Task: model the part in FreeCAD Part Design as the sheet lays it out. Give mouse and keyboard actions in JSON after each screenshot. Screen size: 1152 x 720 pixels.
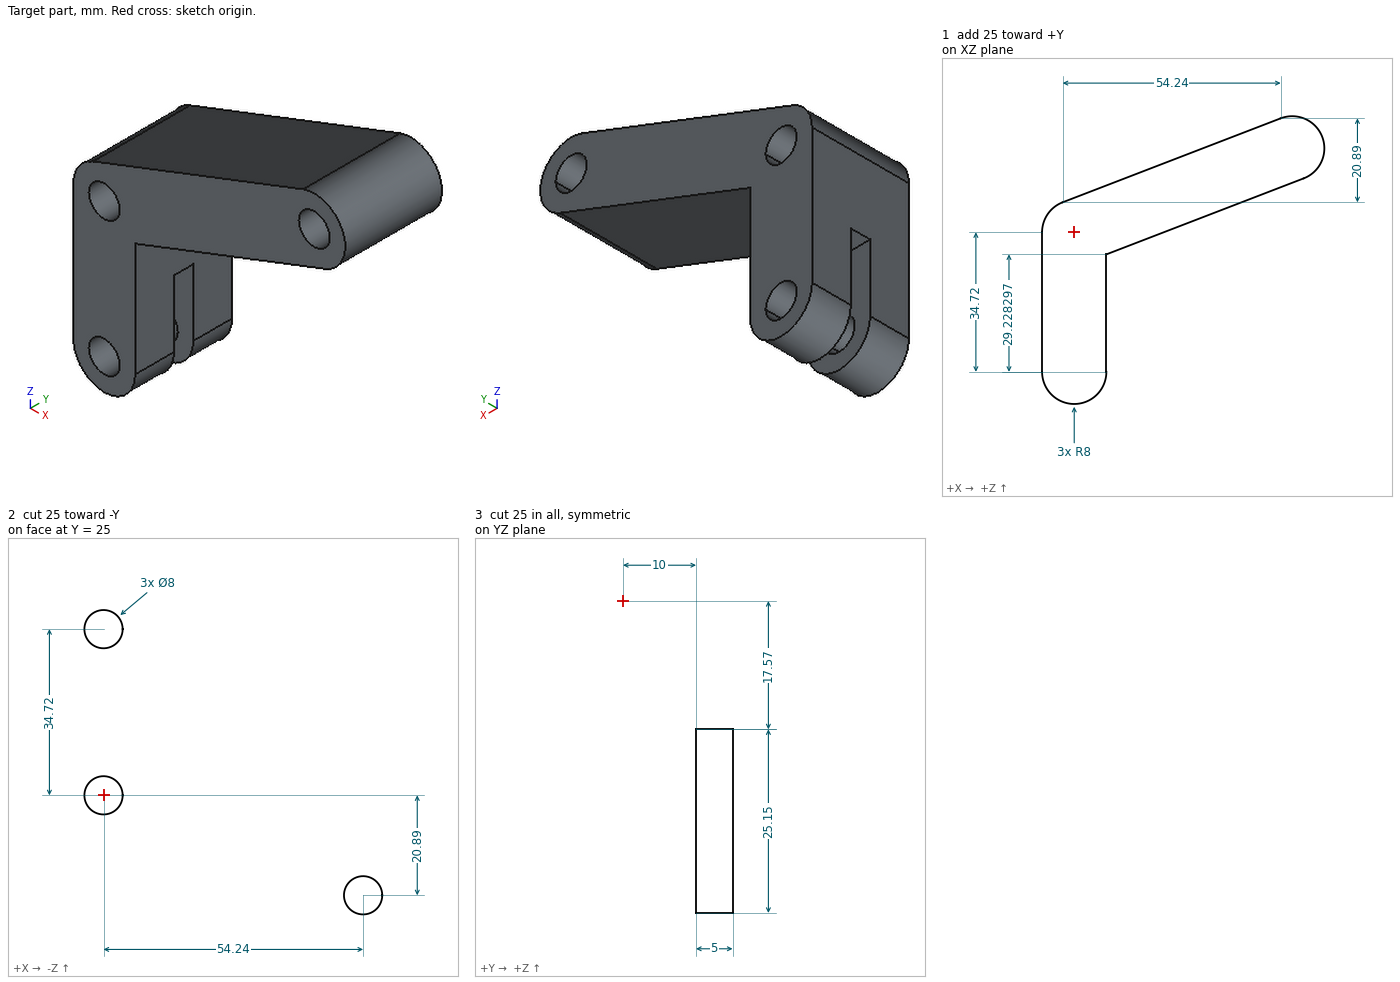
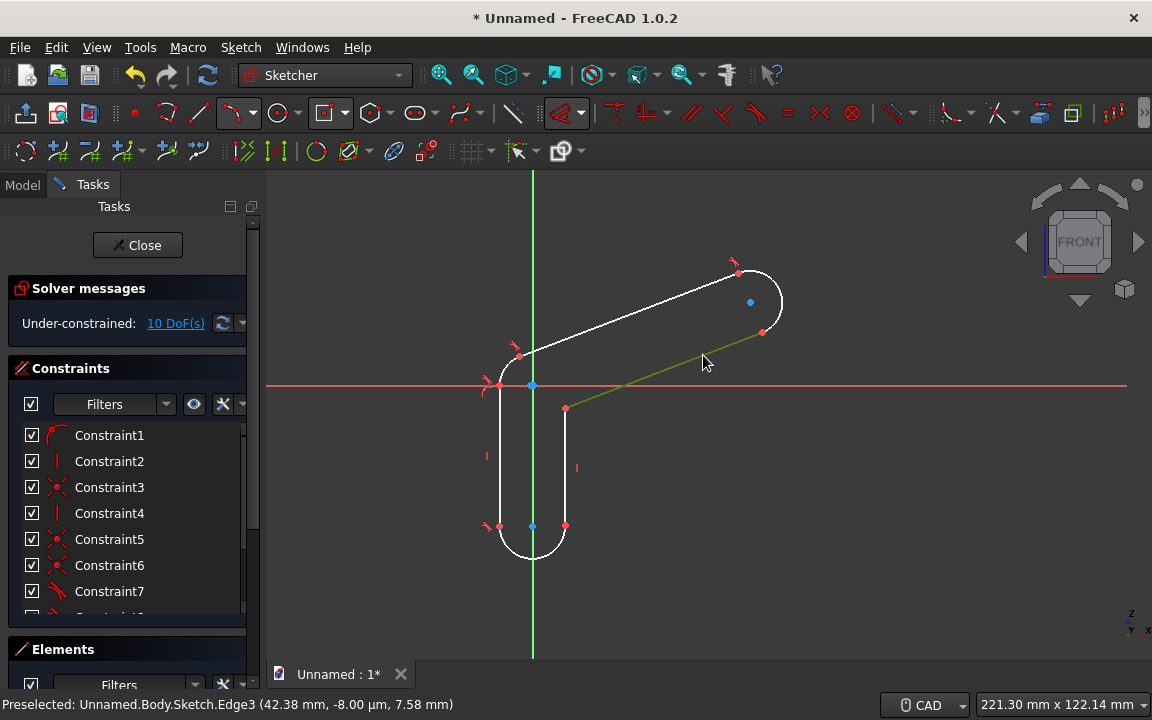
{"action": "left_click", "coordinate": [781, 311]}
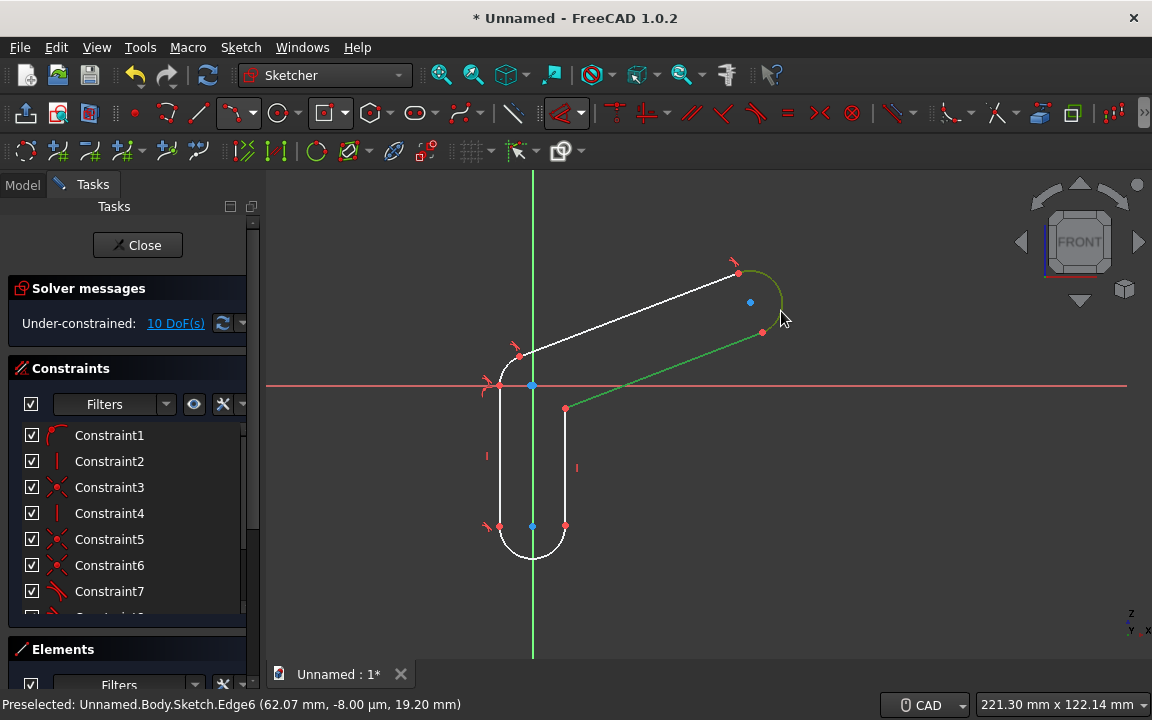
{"action": "left_click", "coordinate": [756, 114]}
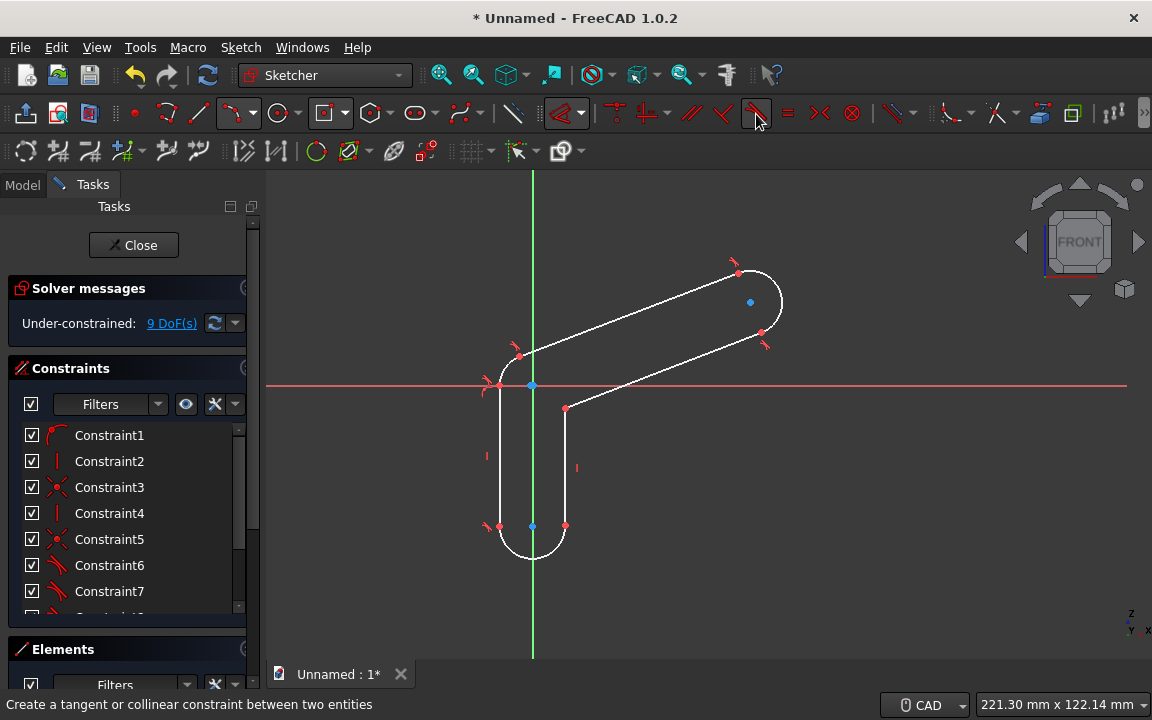
{"action": "left_click", "coordinate": [565, 444]}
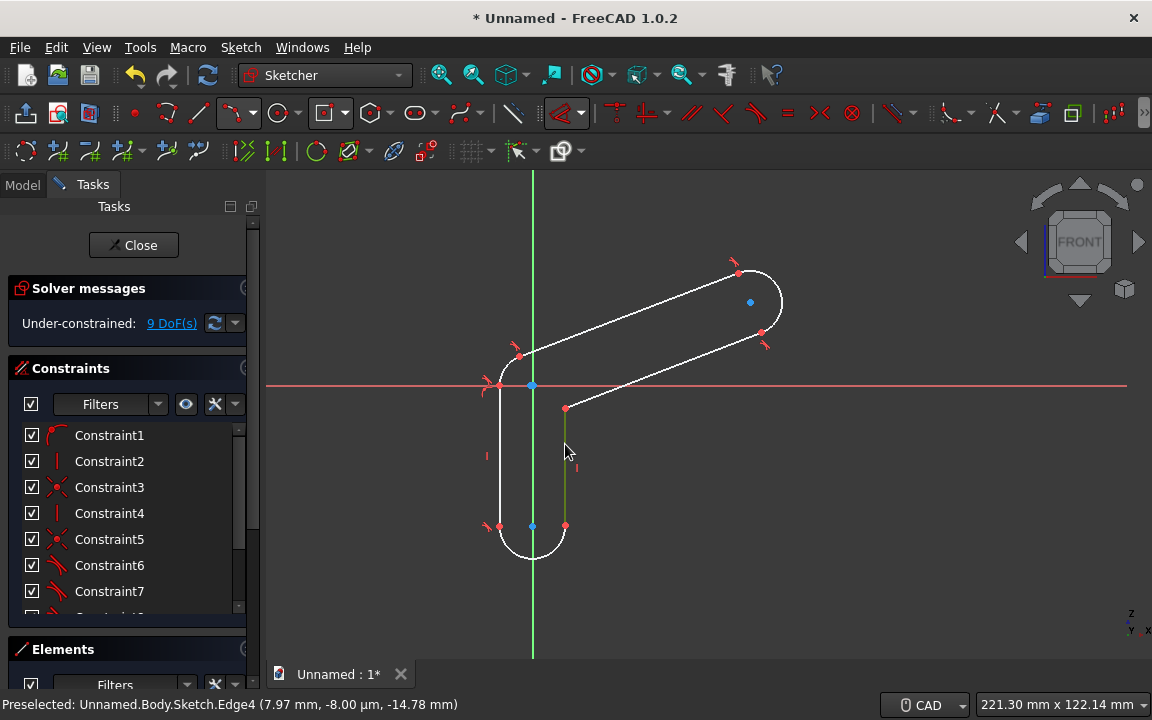
{"action": "left_click", "coordinate": [513, 553]}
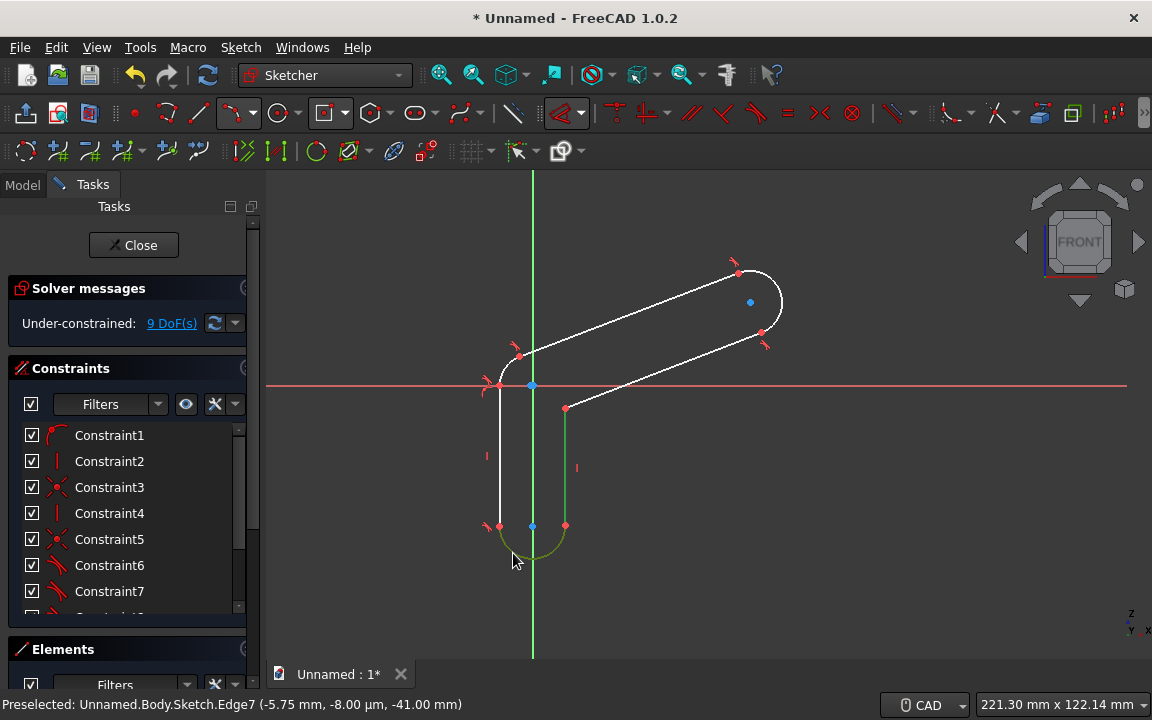
{"action": "left_click", "coordinate": [756, 114]}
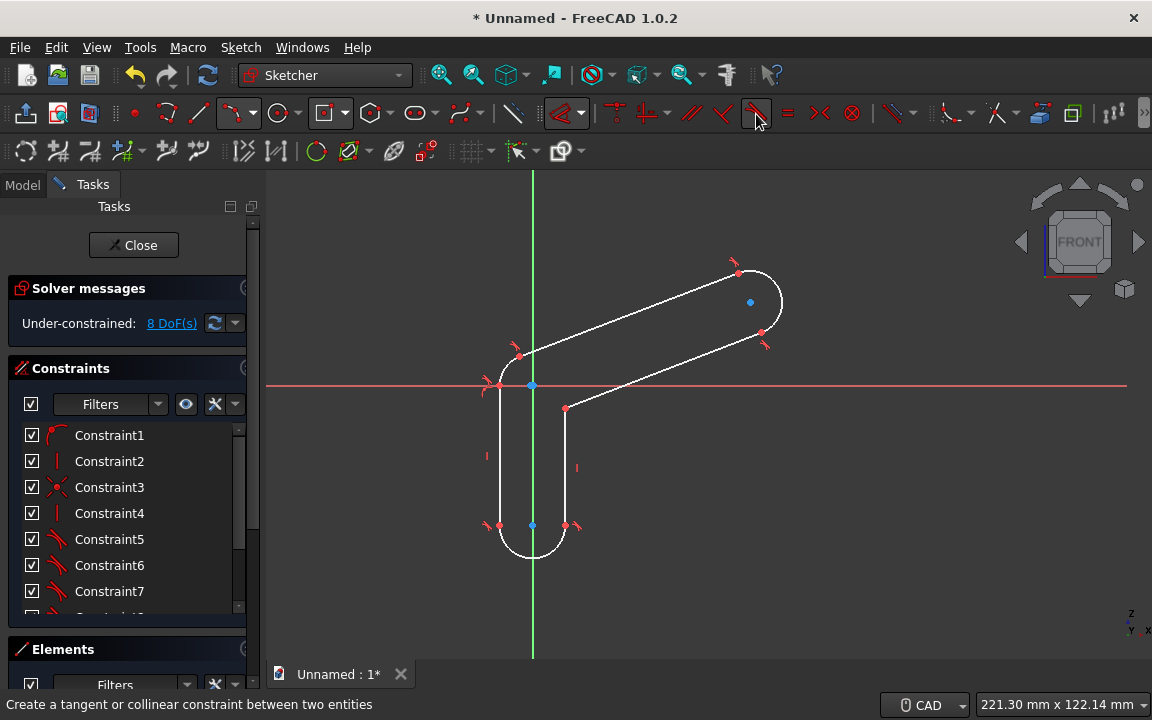
{"action": "scroll", "coordinate": [510, 363], "scroll_direction": "up", "scroll_amount": 2}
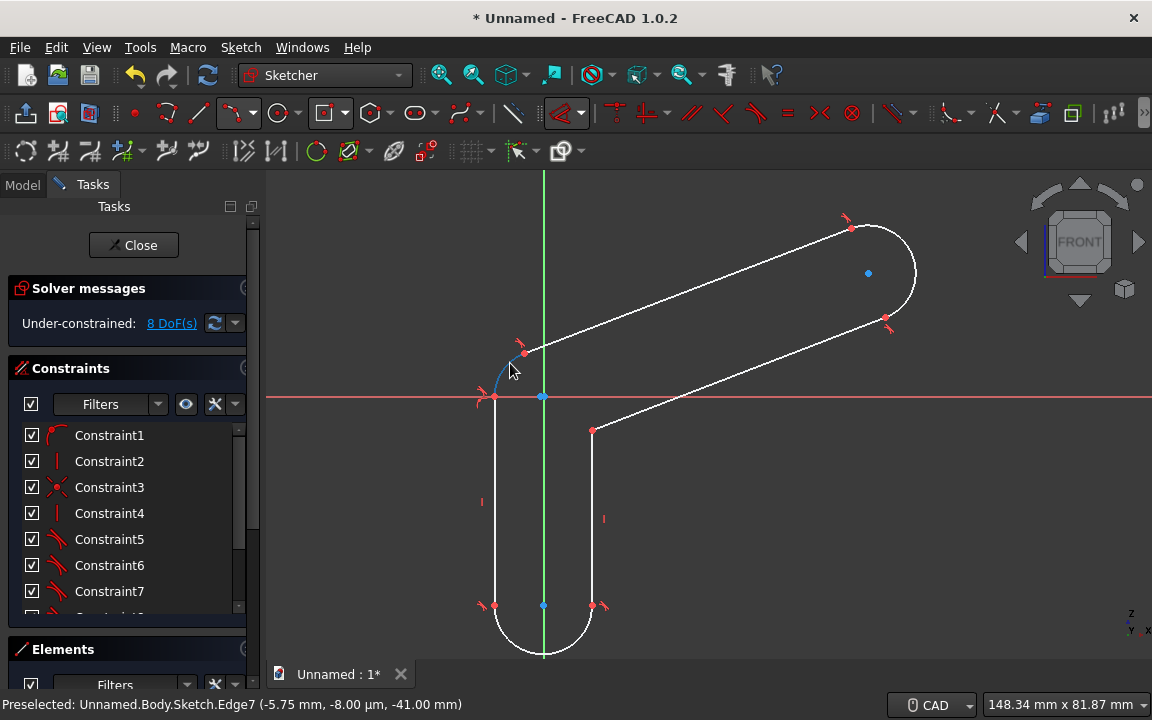
{"action": "left_click", "coordinate": [510, 362]}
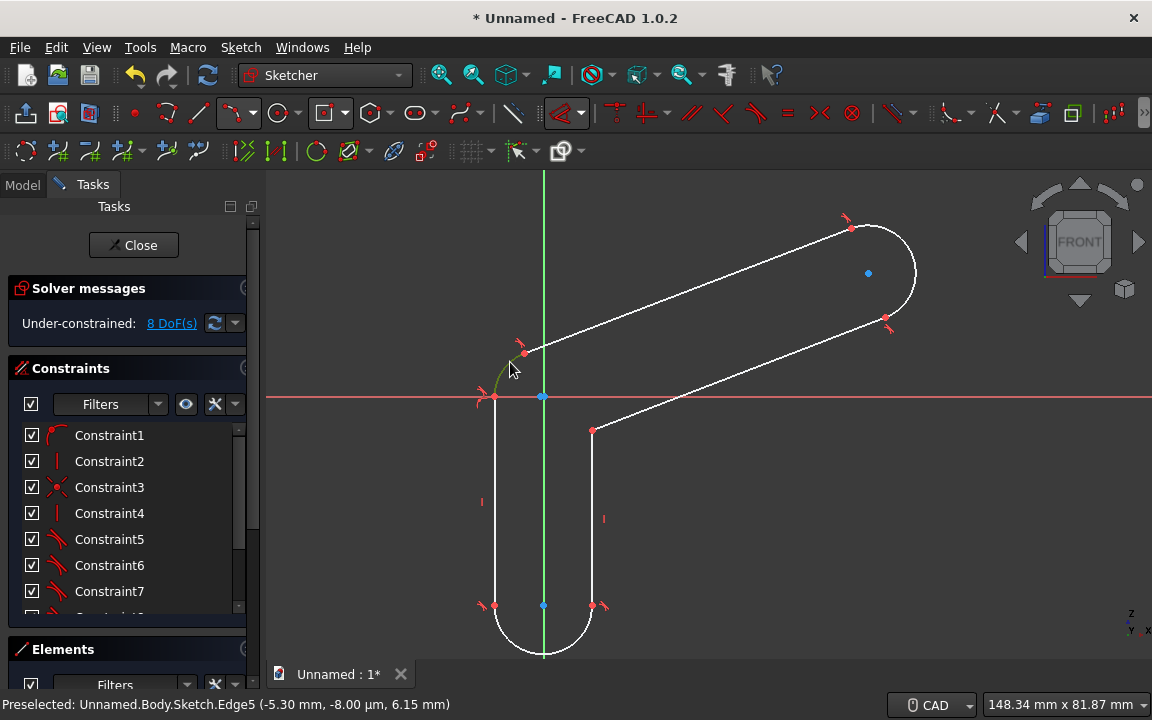
{"action": "left_click", "coordinate": [914, 285]}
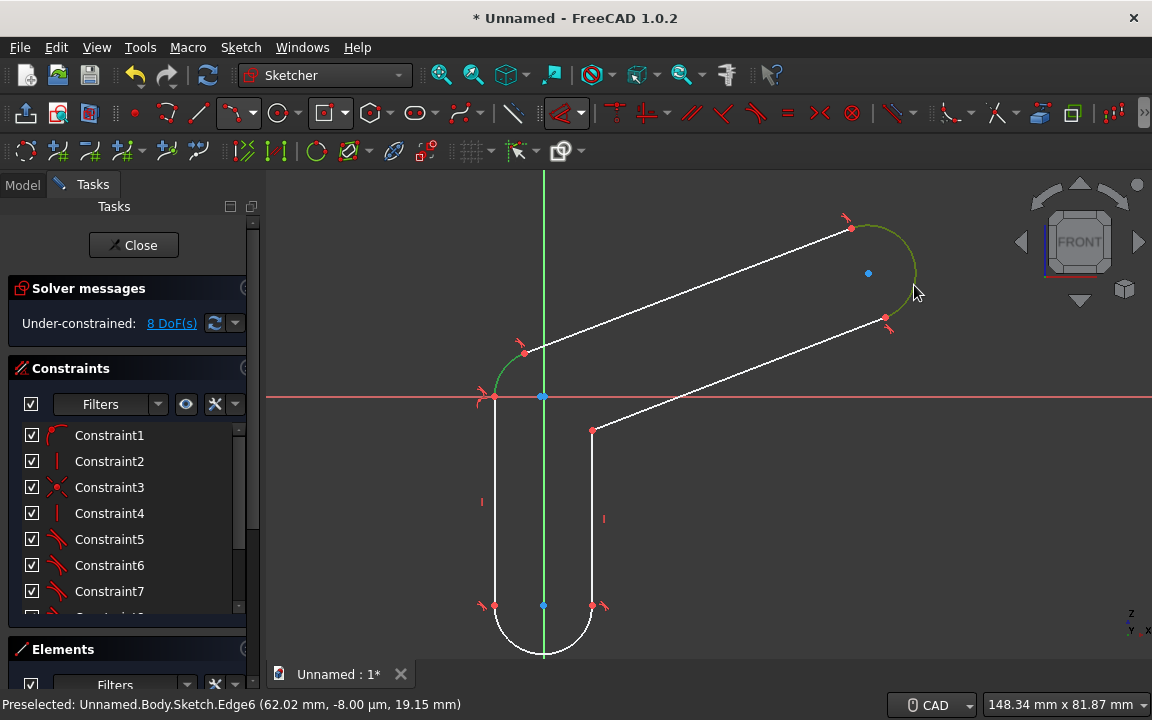
{"action": "scroll", "coordinate": [510, 363], "scroll_direction": "down", "scroll_amount": 2}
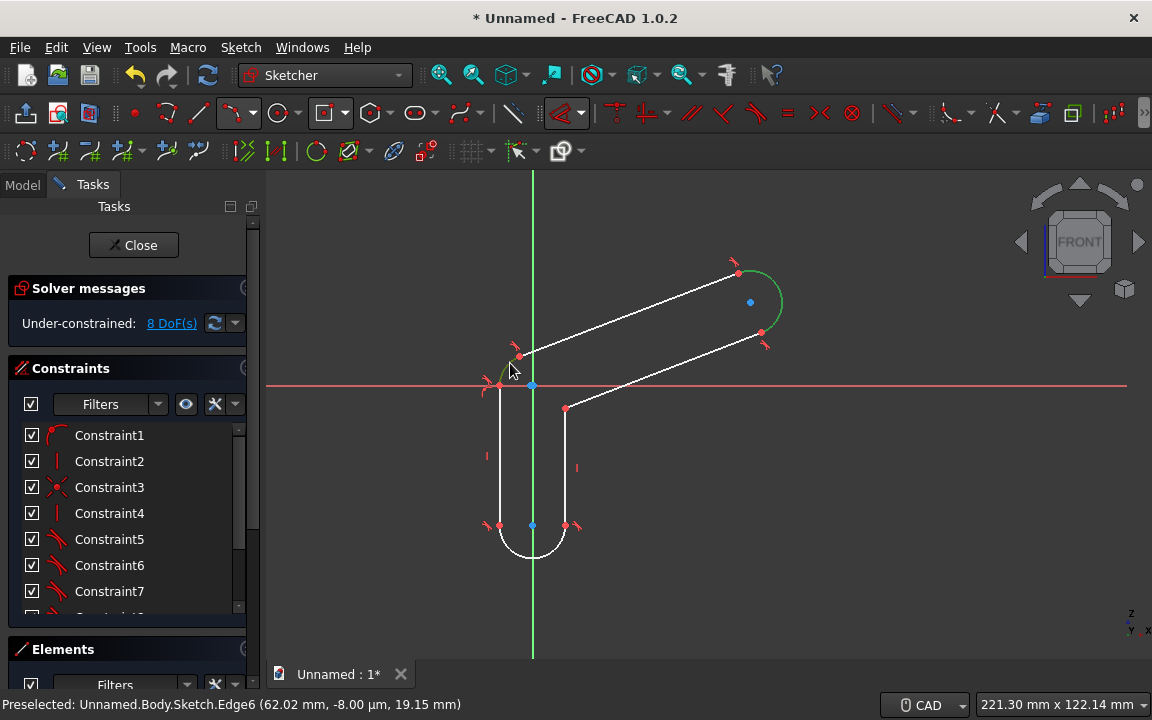
{"action": "left_click", "coordinate": [513, 552]}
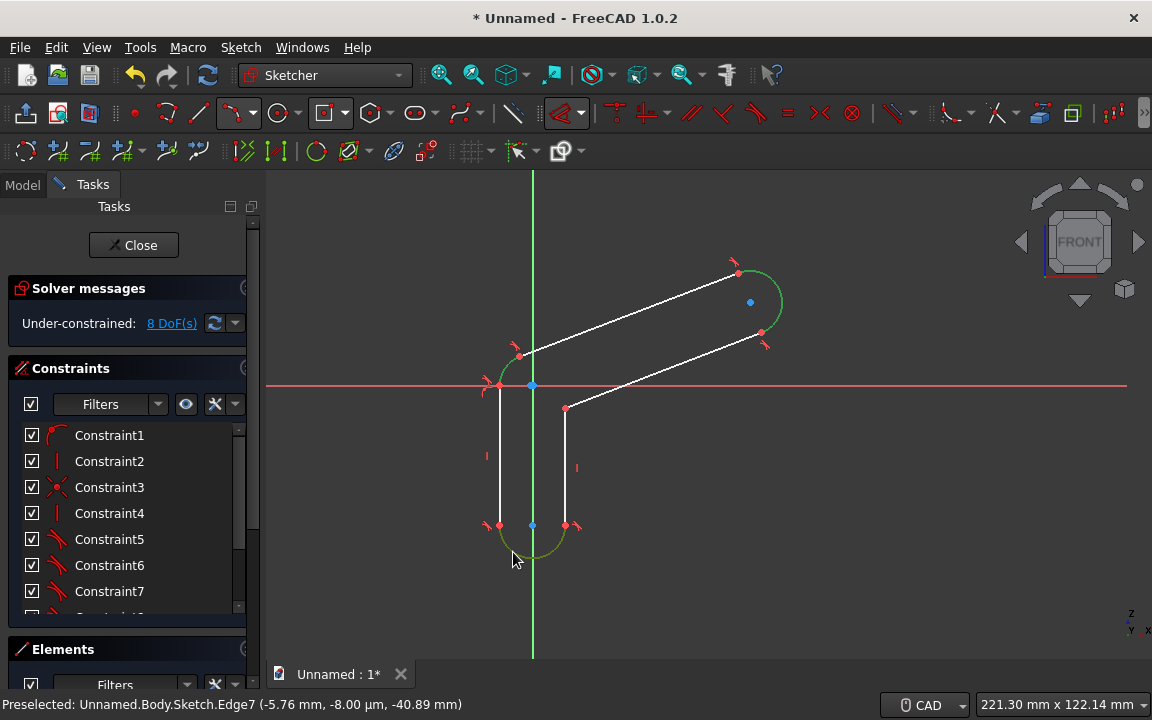
{"action": "left_click", "coordinate": [788, 114]}